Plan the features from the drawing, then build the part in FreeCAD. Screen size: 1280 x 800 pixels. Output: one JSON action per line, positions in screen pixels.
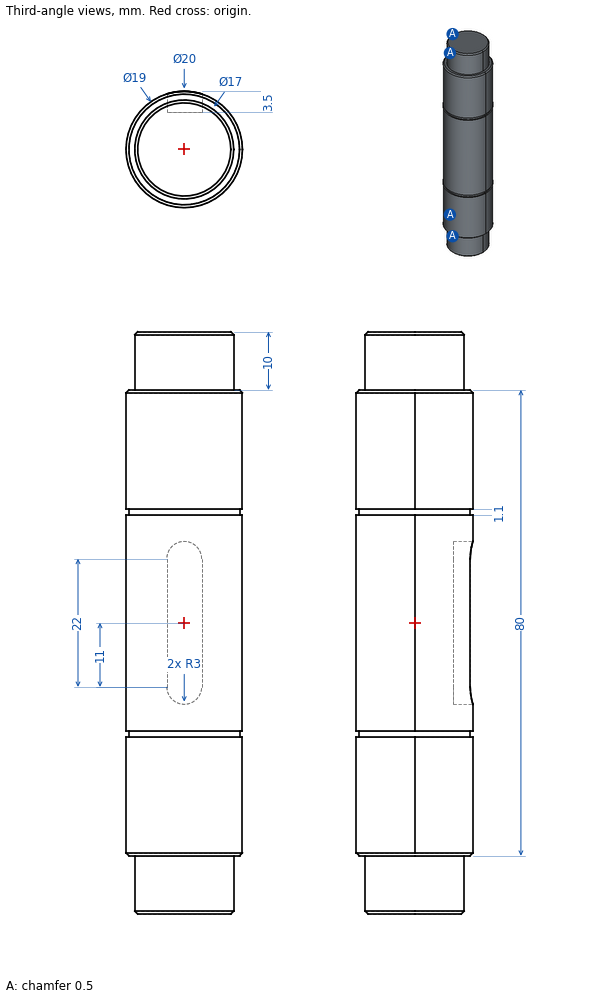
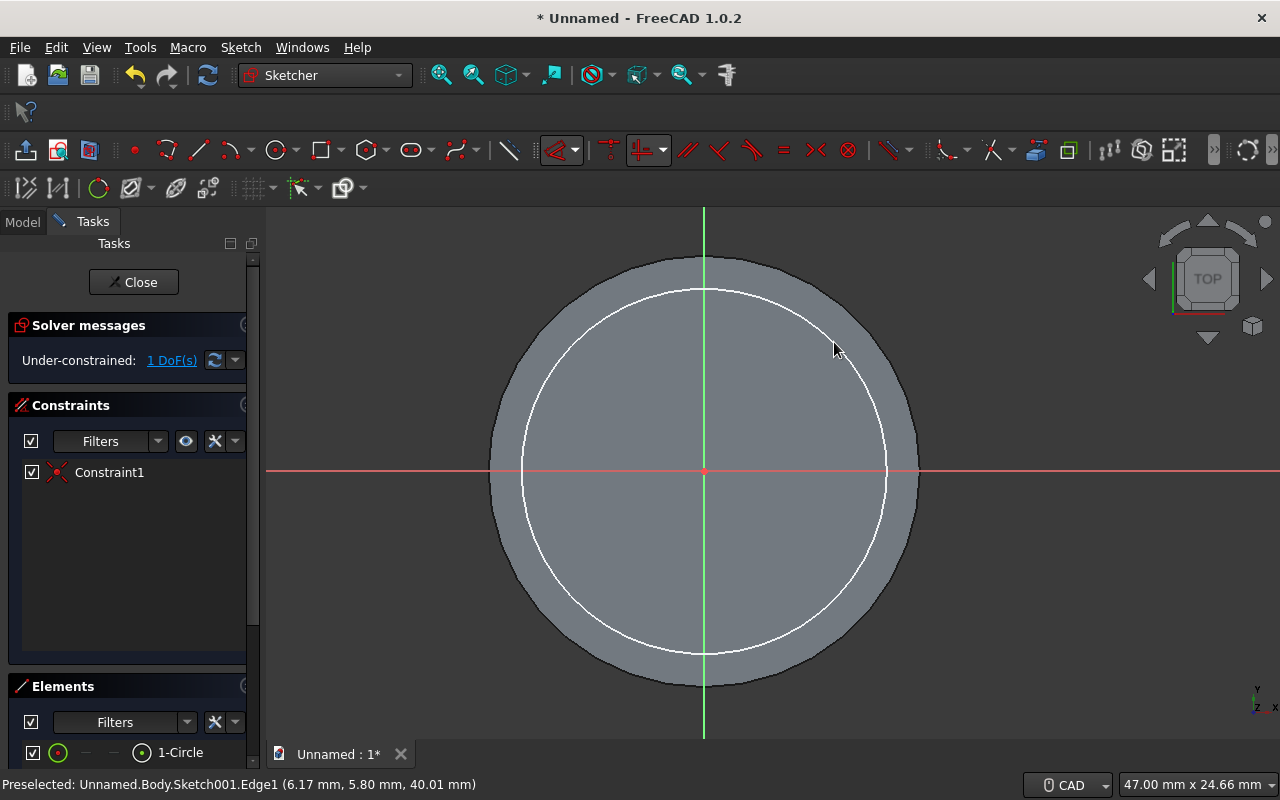
{"action": "key", "text": "d"}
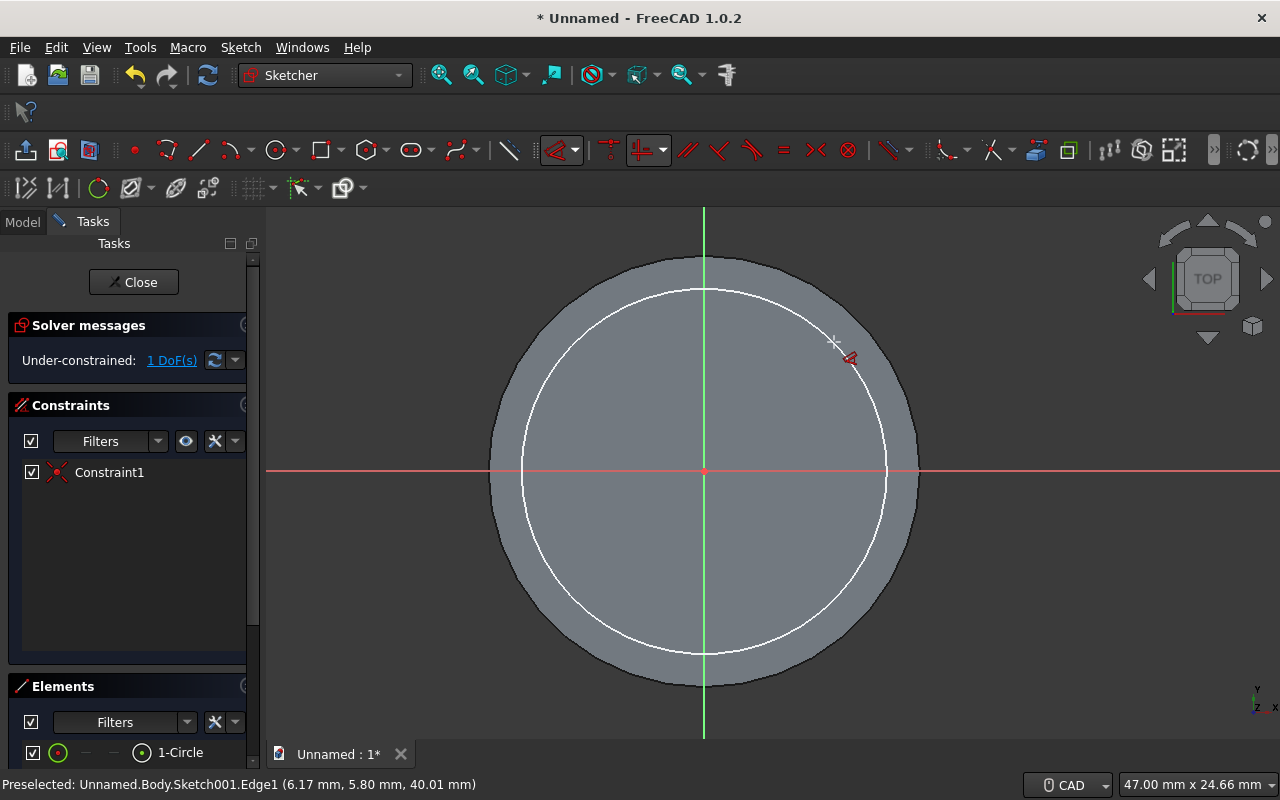
{"action": "left_click", "coordinate": [833, 342]}
{"action": "left_click", "coordinate": [856, 319]}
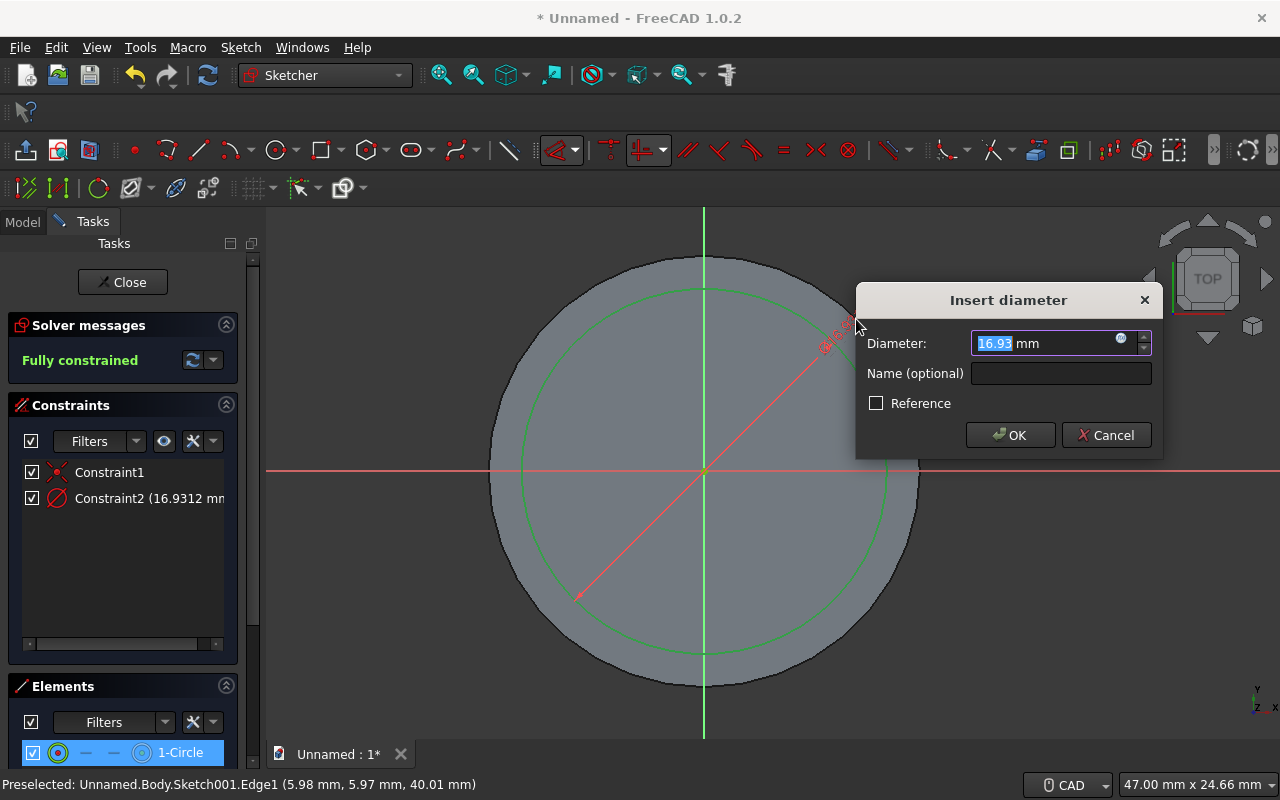
{"action": "type", "text": "17"}
{"action": "key", "text": "Return"}
{"action": "key", "text": "Escape"}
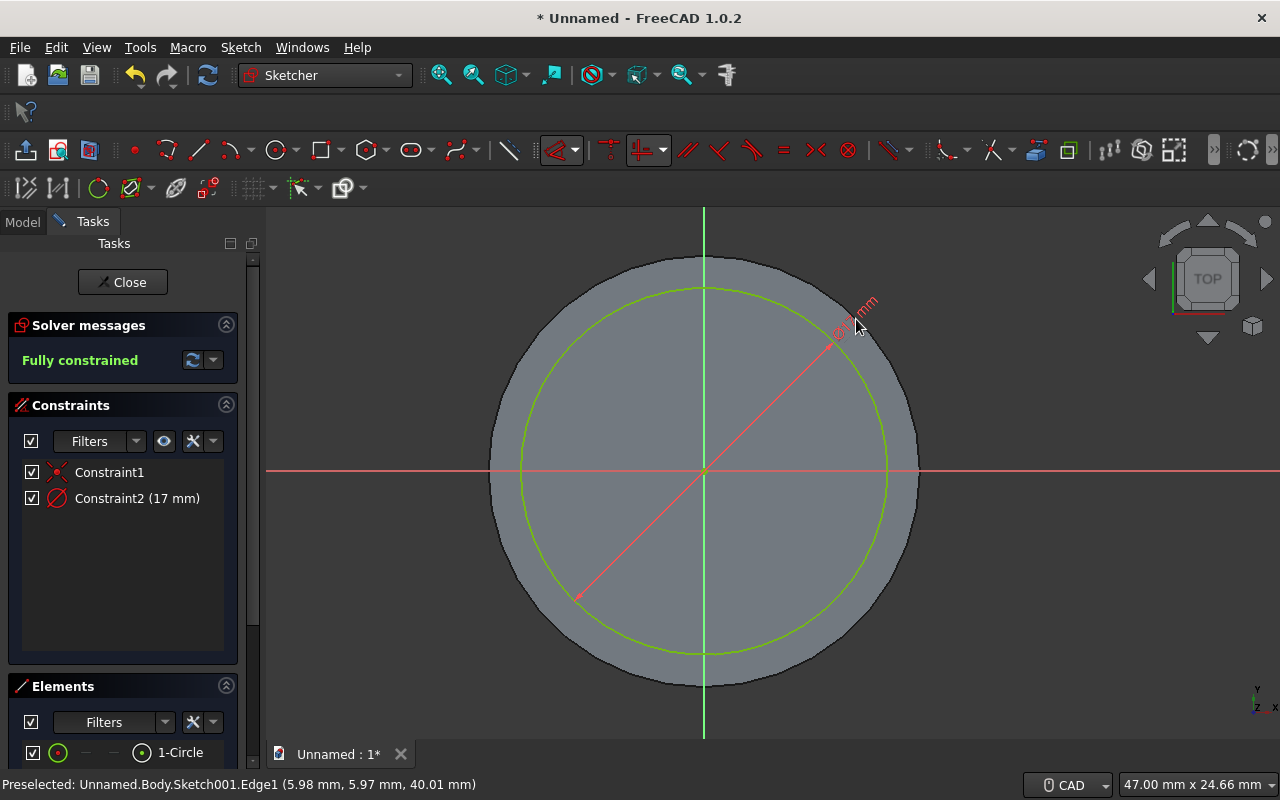
{"action": "left_click", "coordinate": [123, 282]}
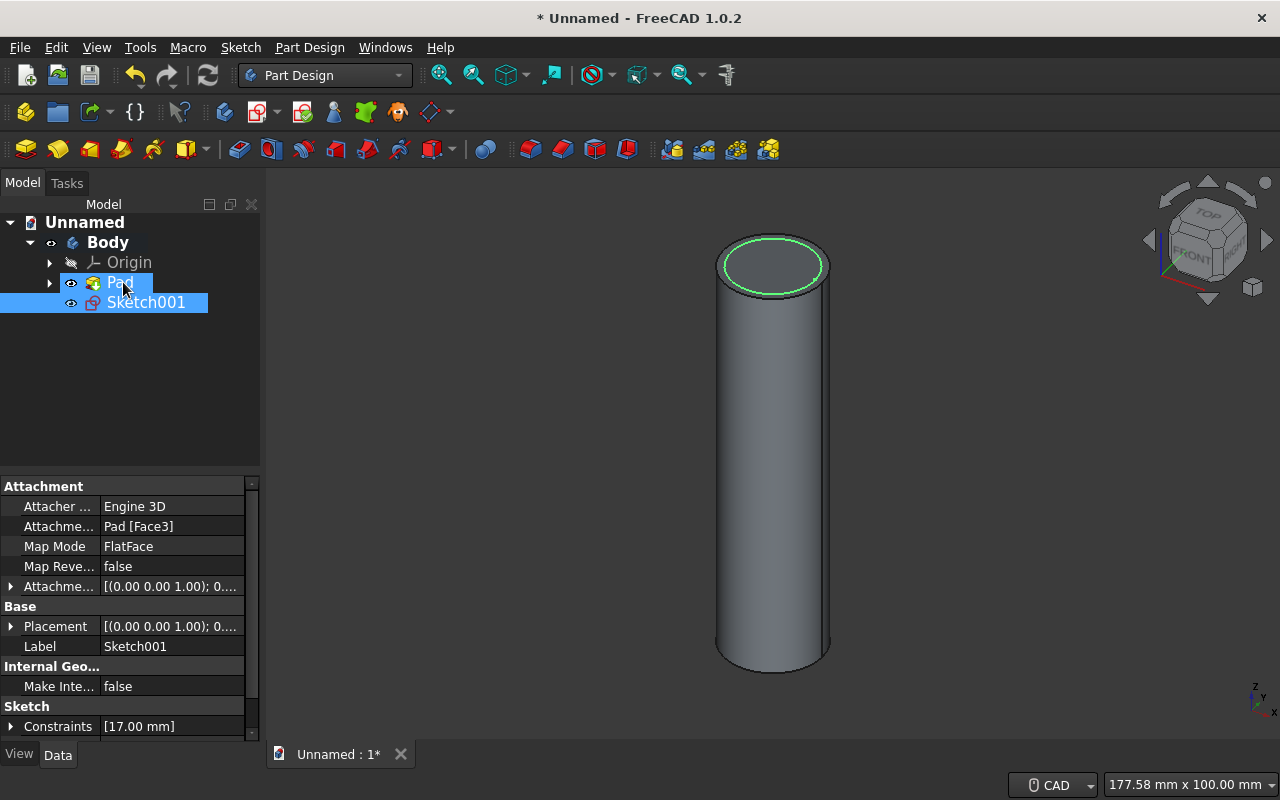
{"action": "left_click", "coordinate": [26, 150]}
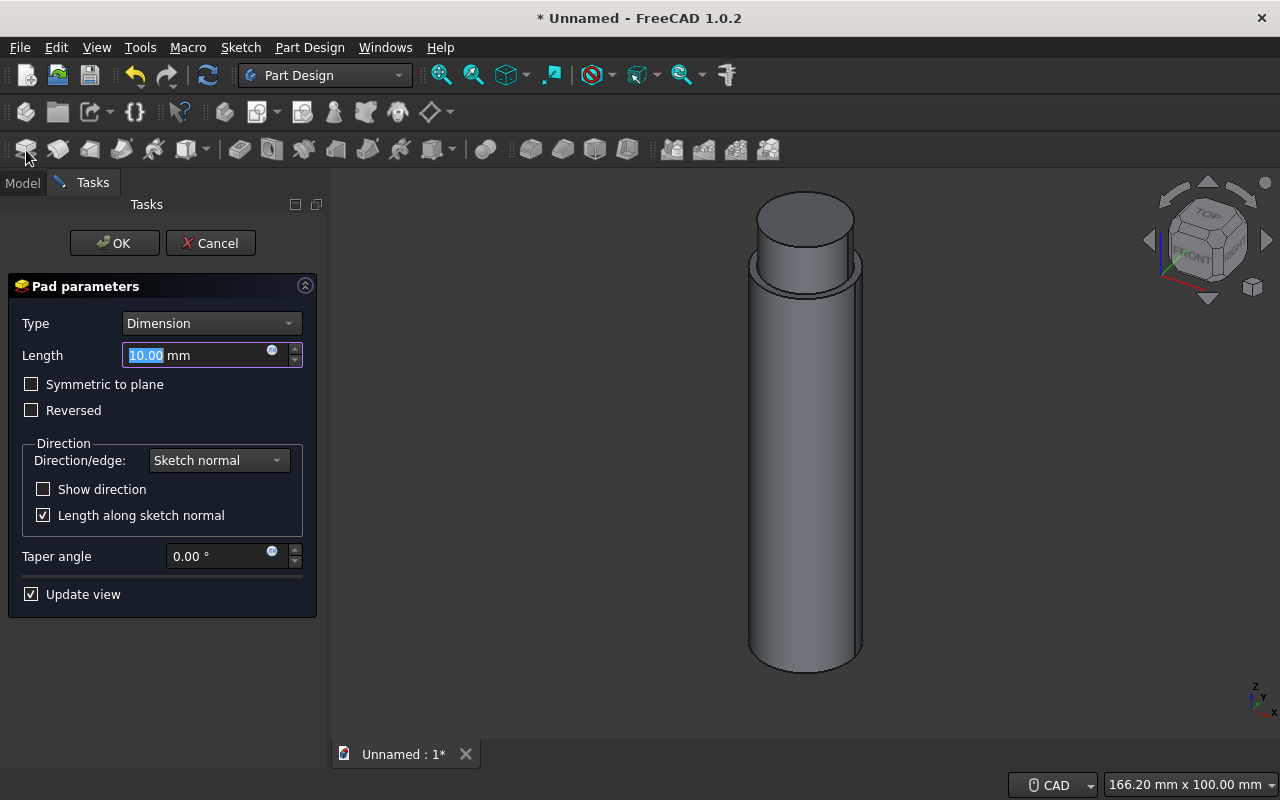
{"action": "type", "text": "10"}
{"action": "key", "text": "Tab"}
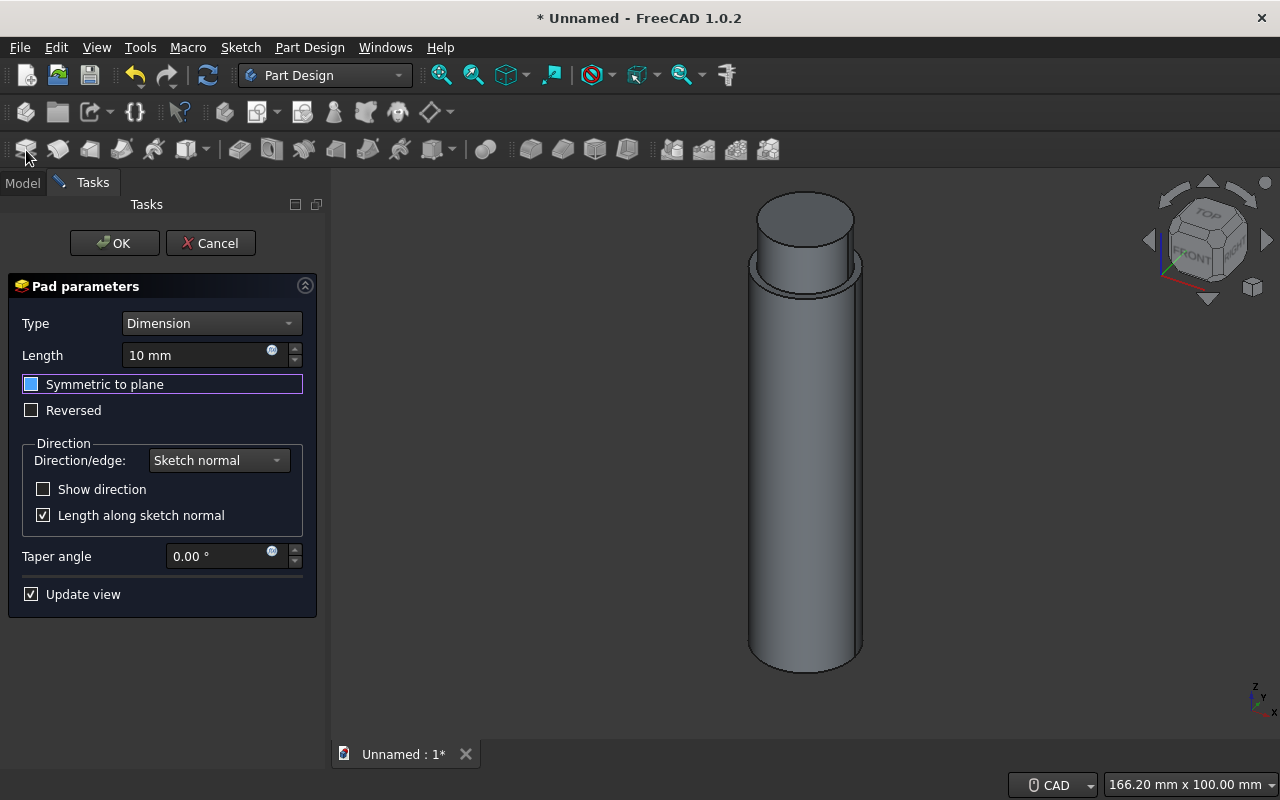
{"action": "left_click", "coordinate": [115, 243]}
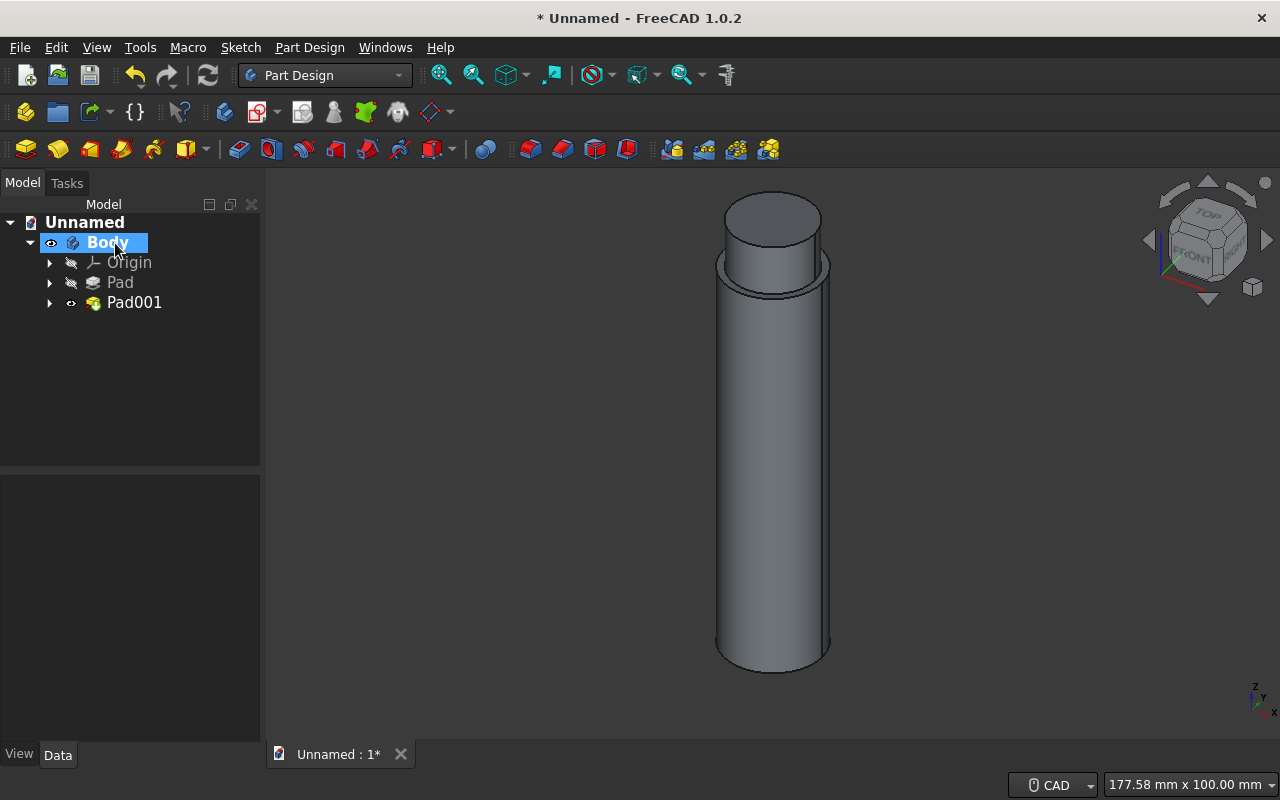
{"action": "left_click", "coordinate": [50, 263]}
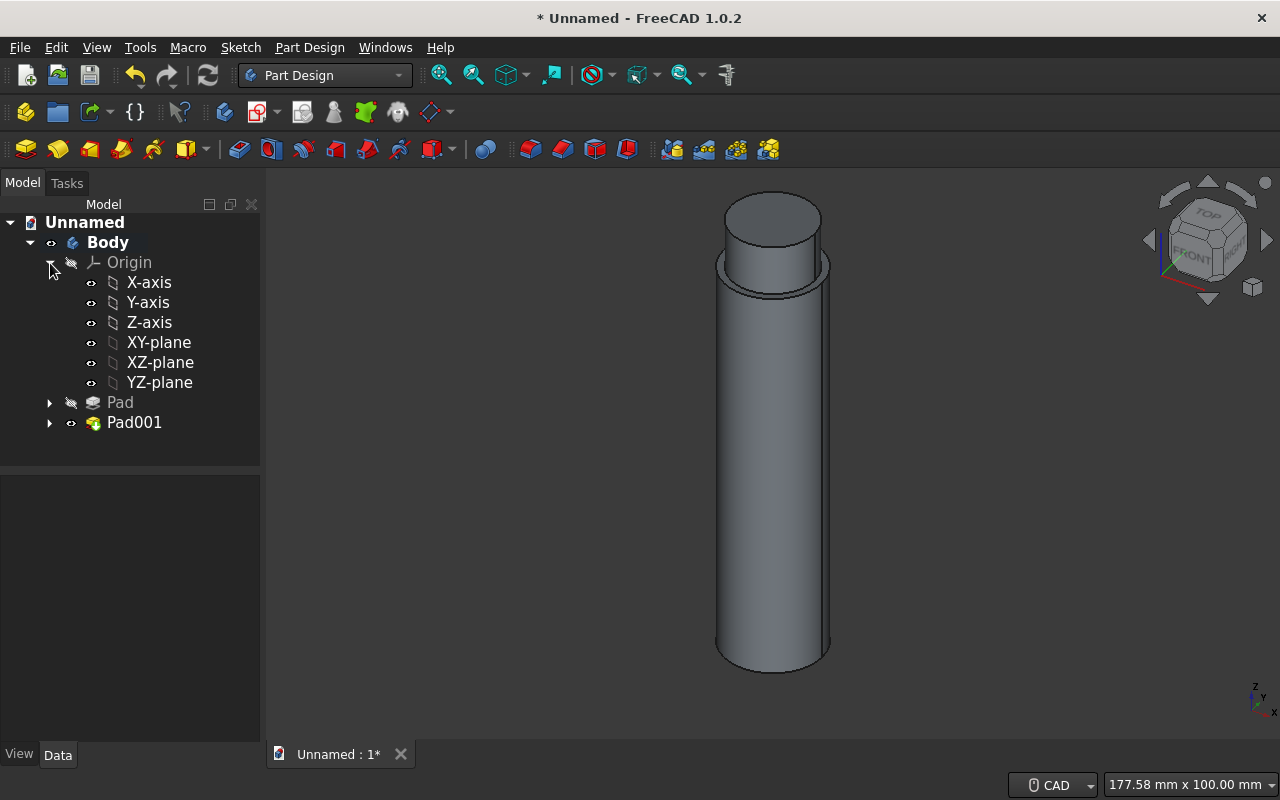
{"action": "left_click", "coordinate": [136, 343]}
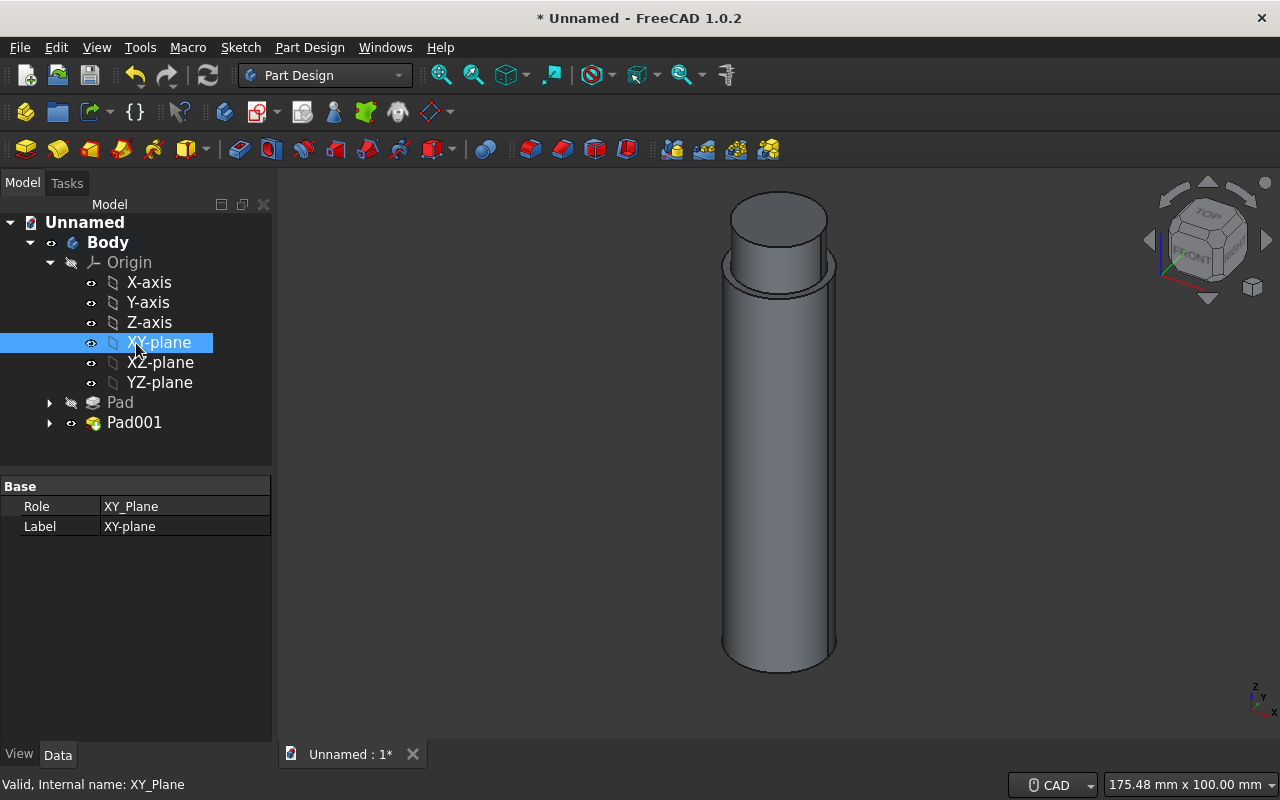
{"action": "left_click", "coordinate": [430, 112]}